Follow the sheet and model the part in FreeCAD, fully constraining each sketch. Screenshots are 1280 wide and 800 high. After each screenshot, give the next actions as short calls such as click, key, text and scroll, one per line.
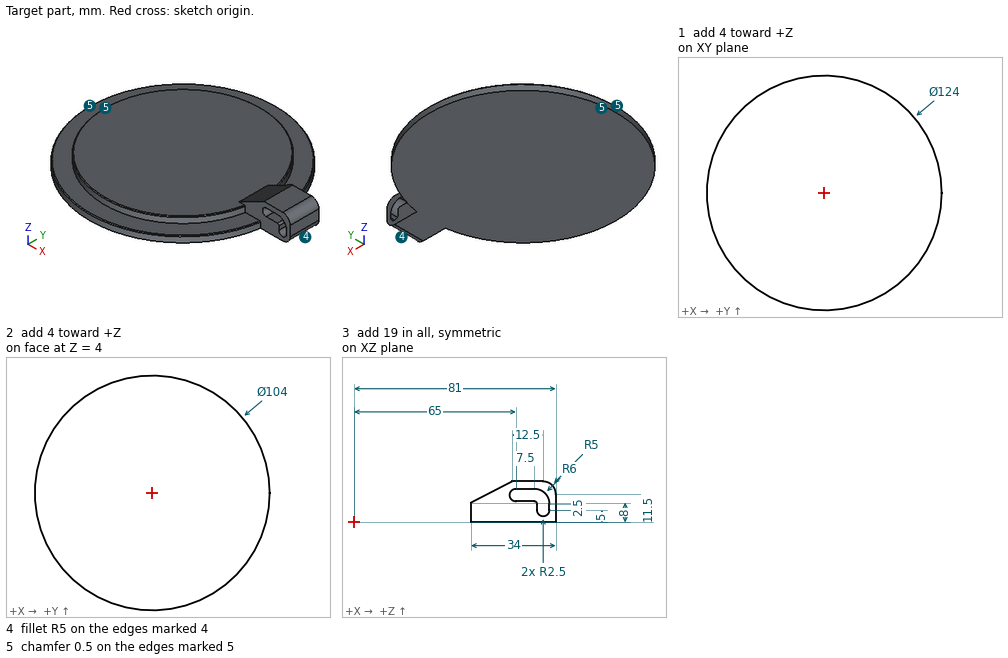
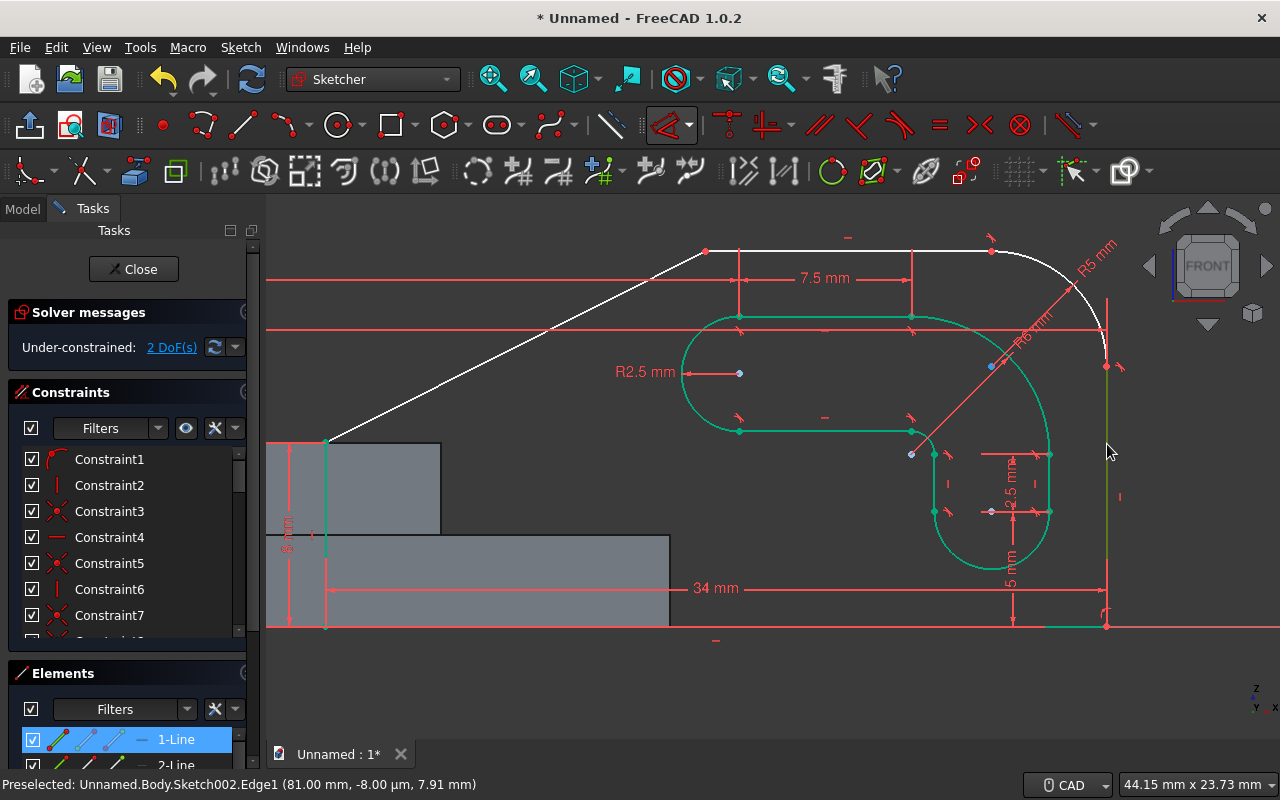
key(i)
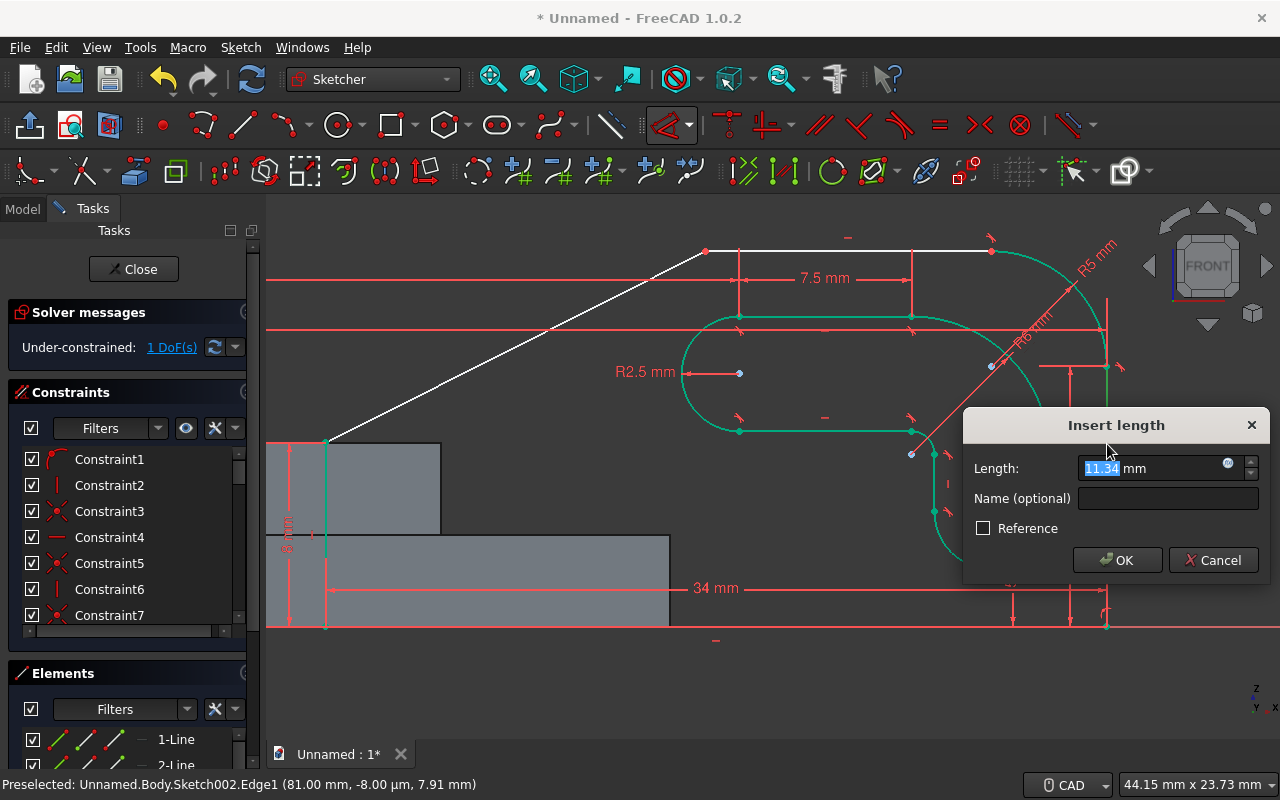
text(11.5)
key(Return)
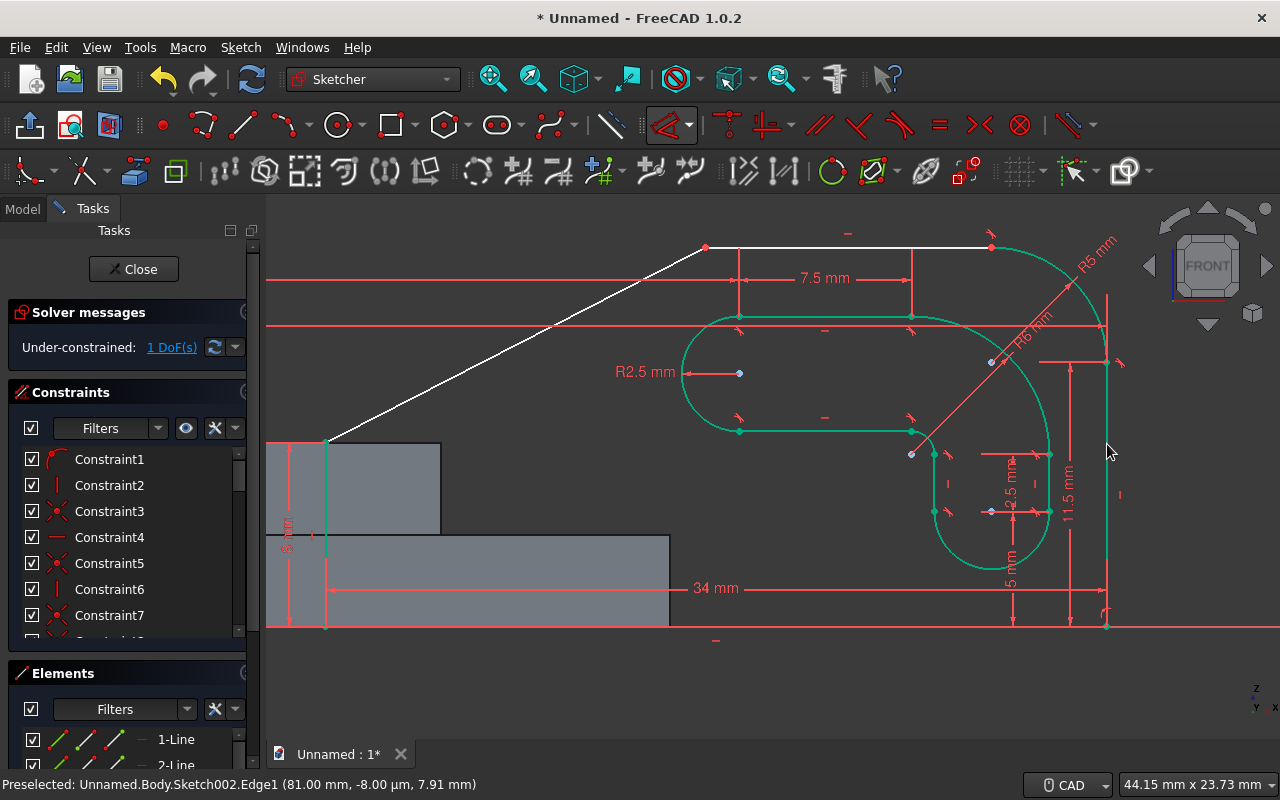
click(791, 248)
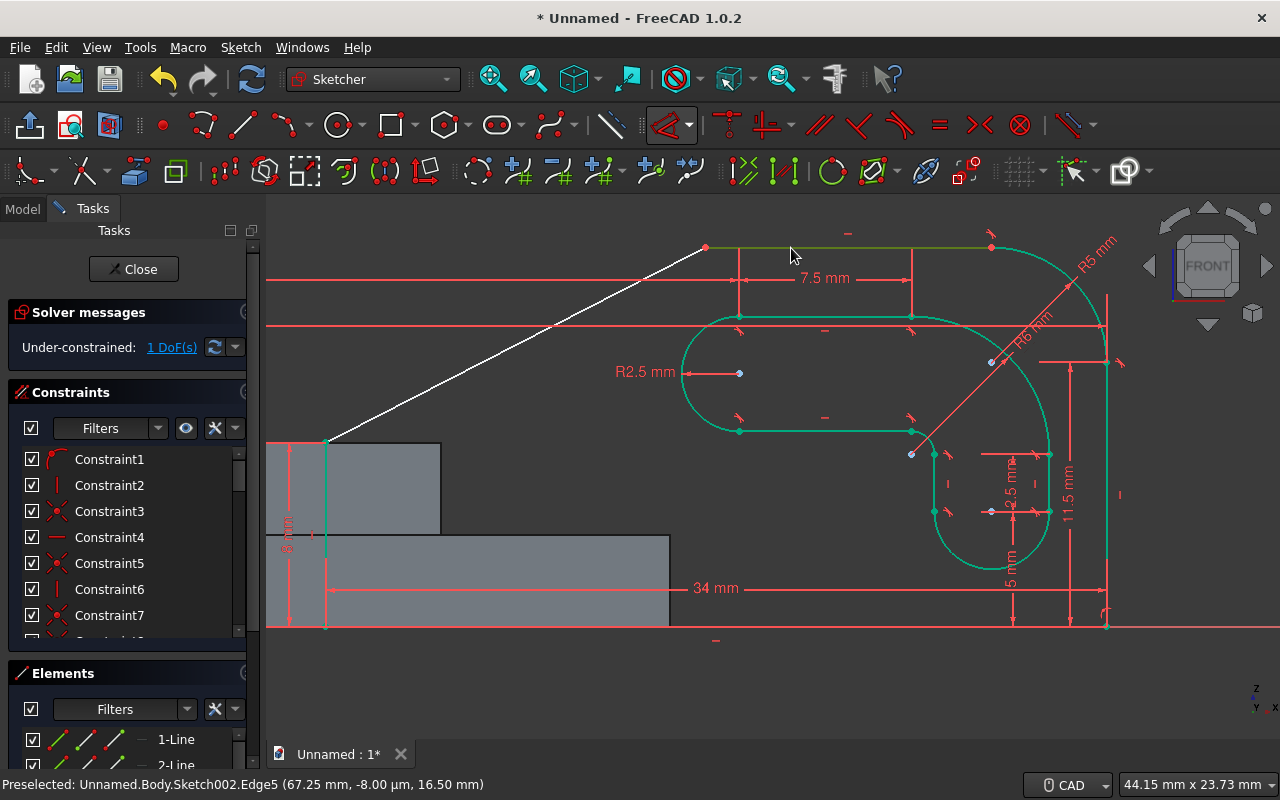
click(692, 126)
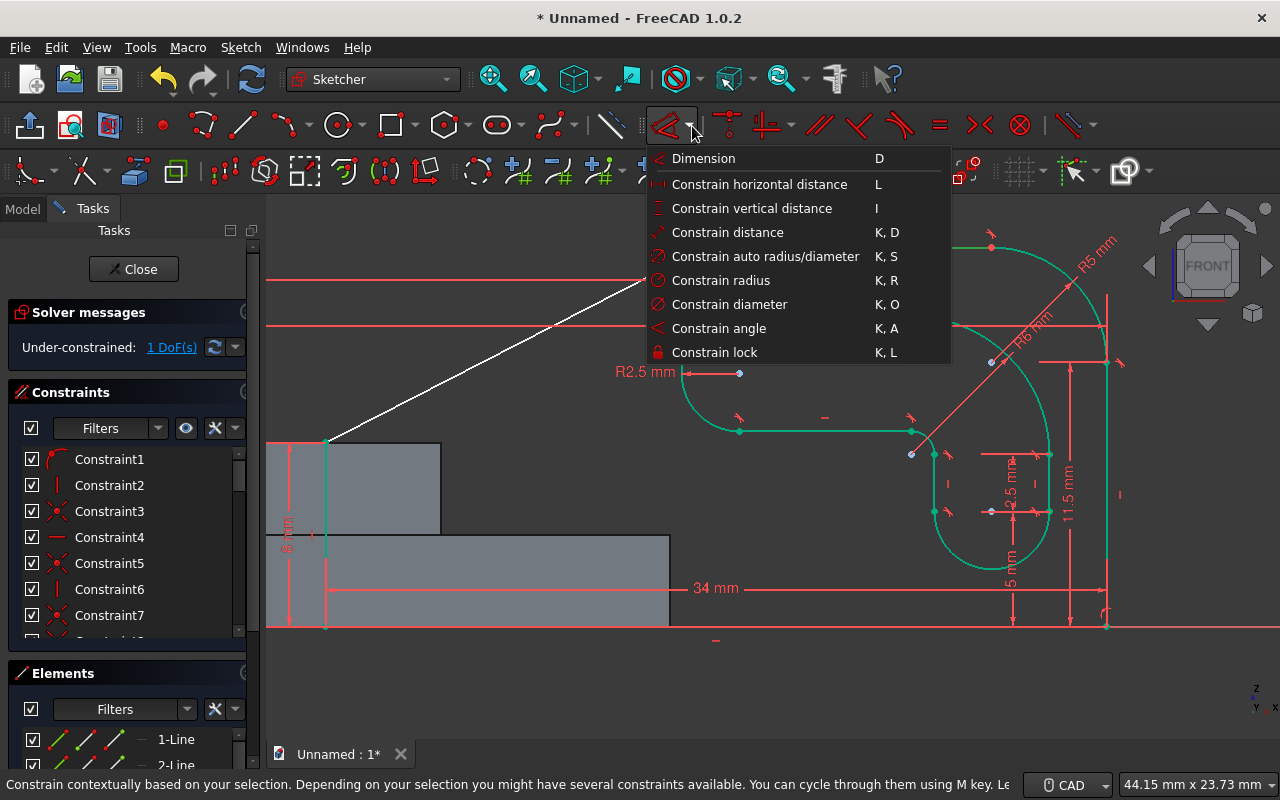
click(799, 184)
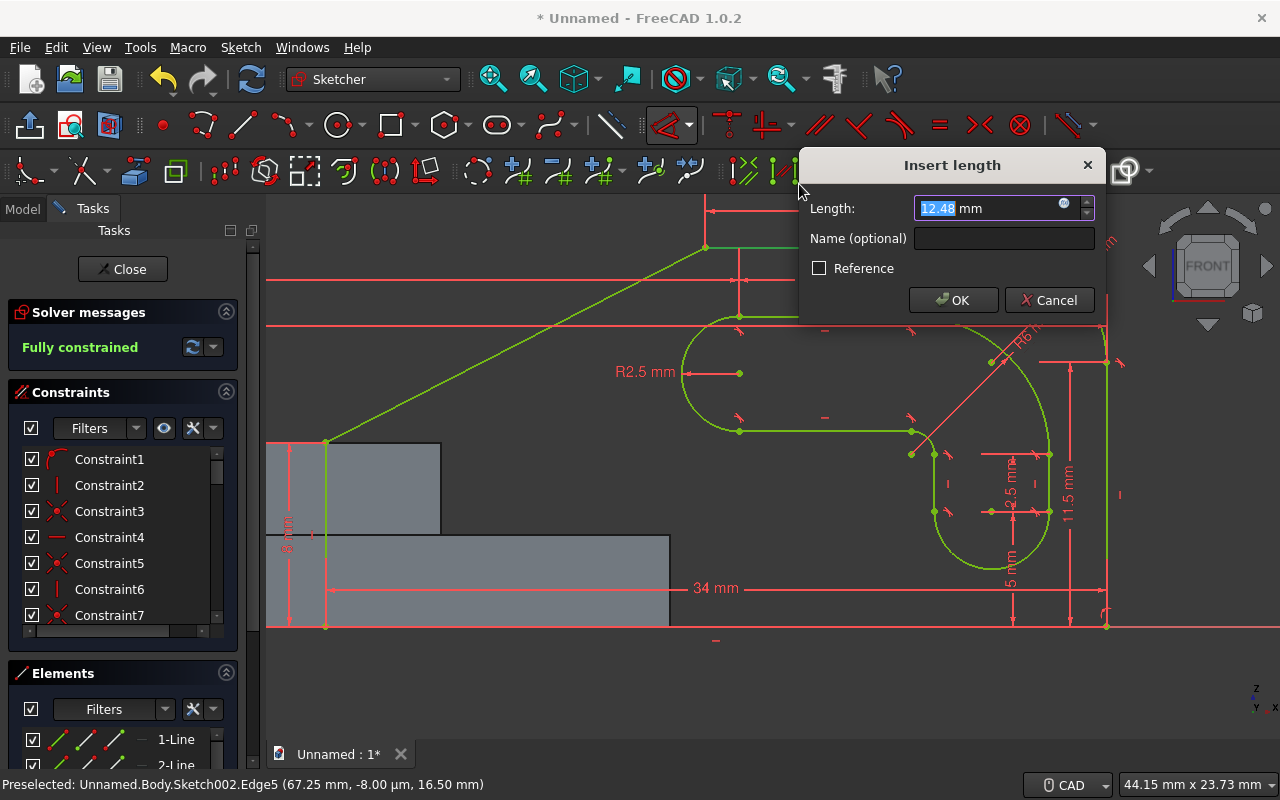
text(12.5)
key(Return)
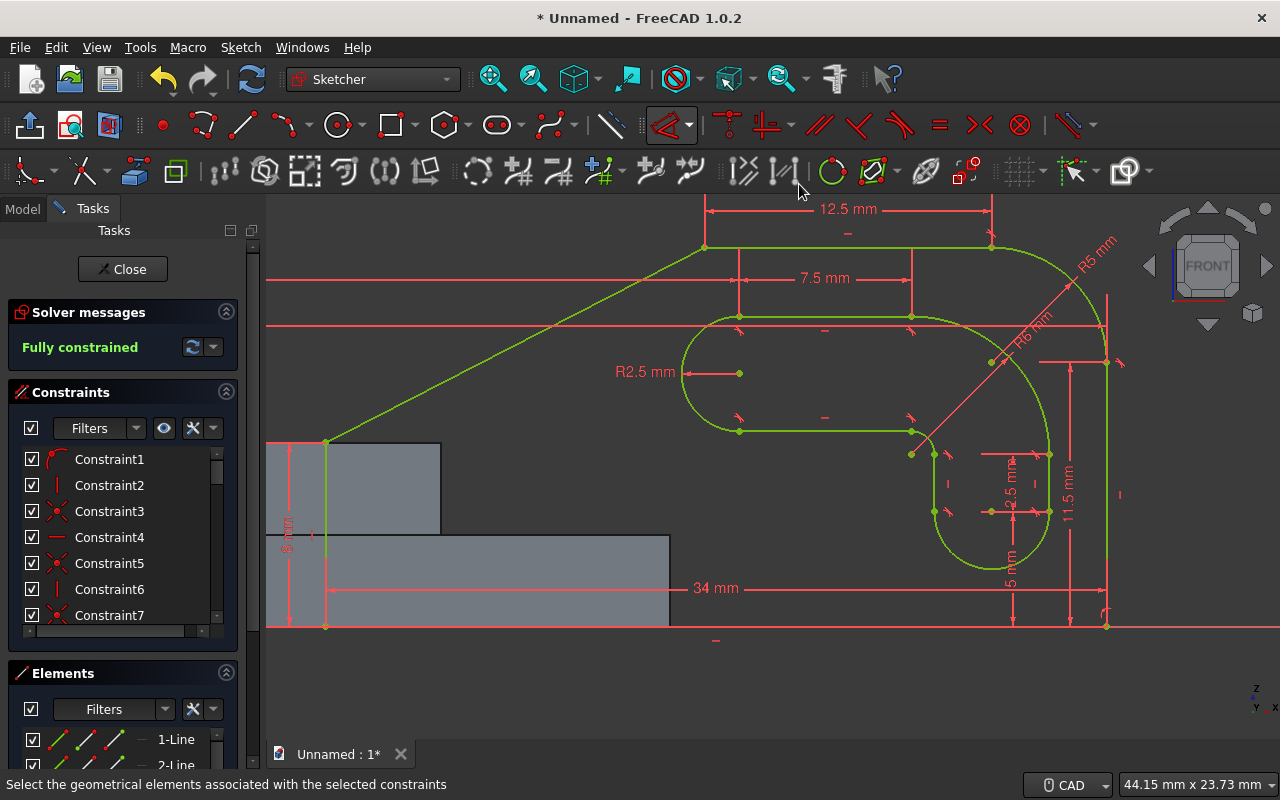
click(123, 269)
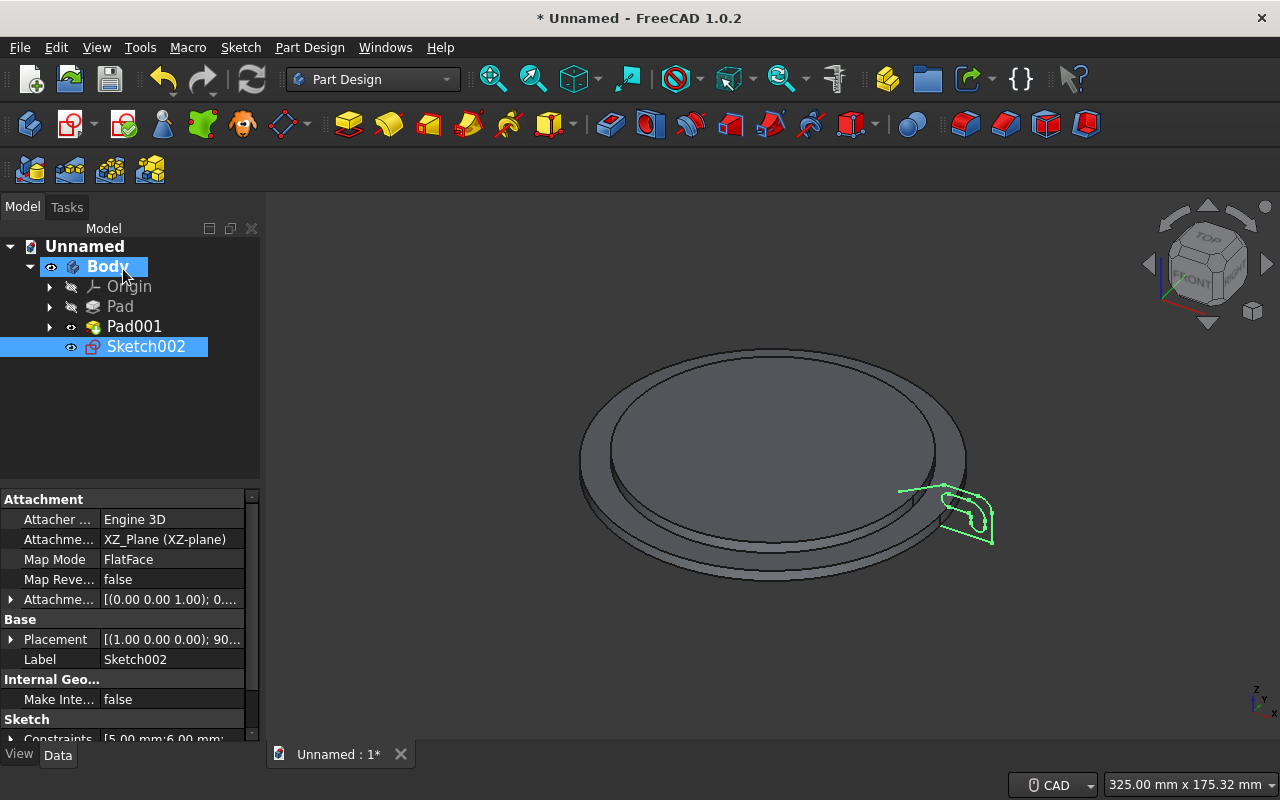
click(350, 124)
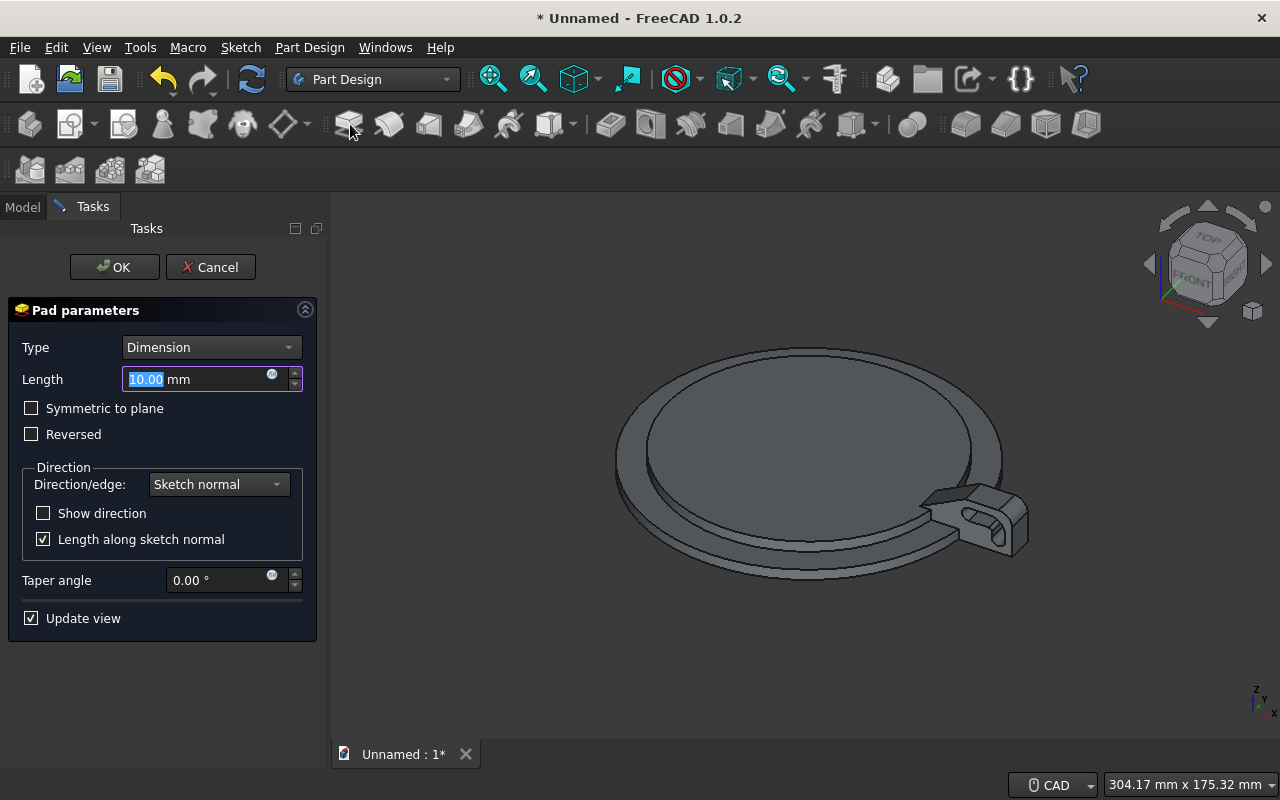
text(19)
key(Tab)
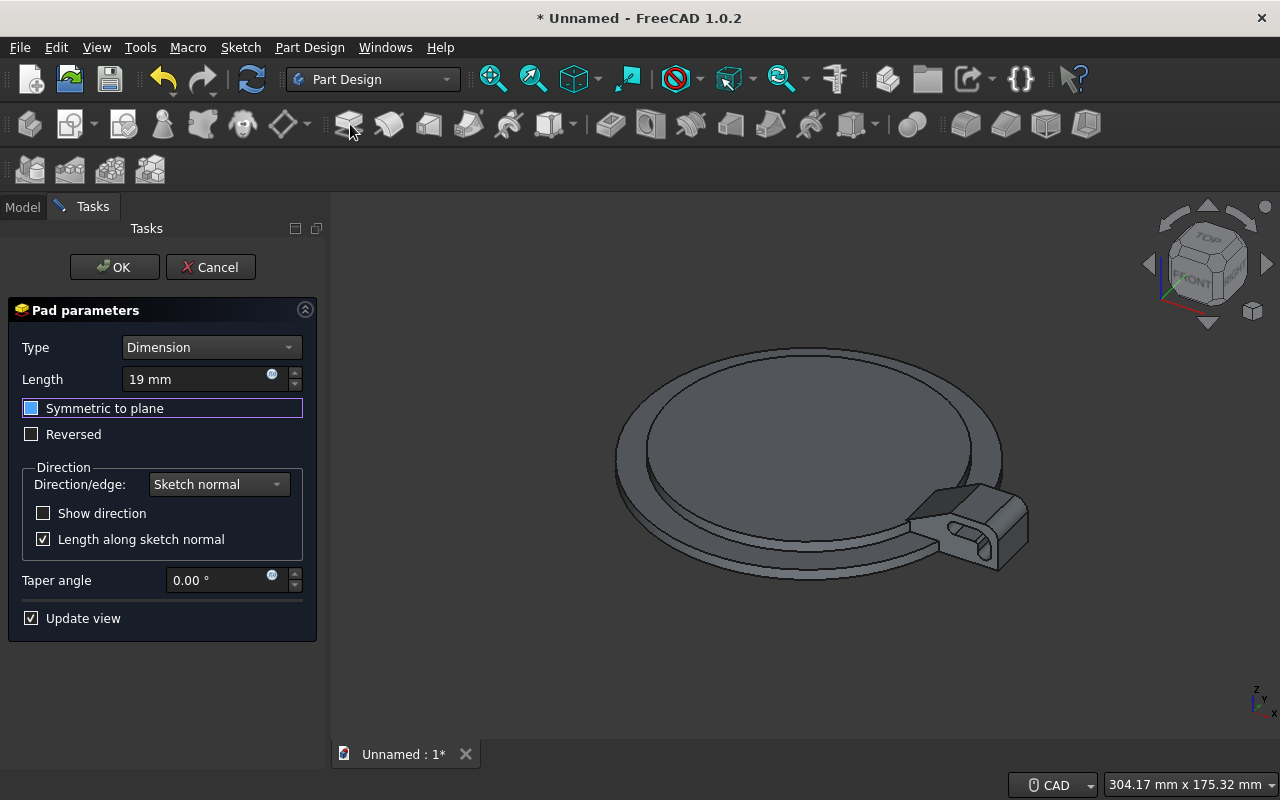
click(30, 408)